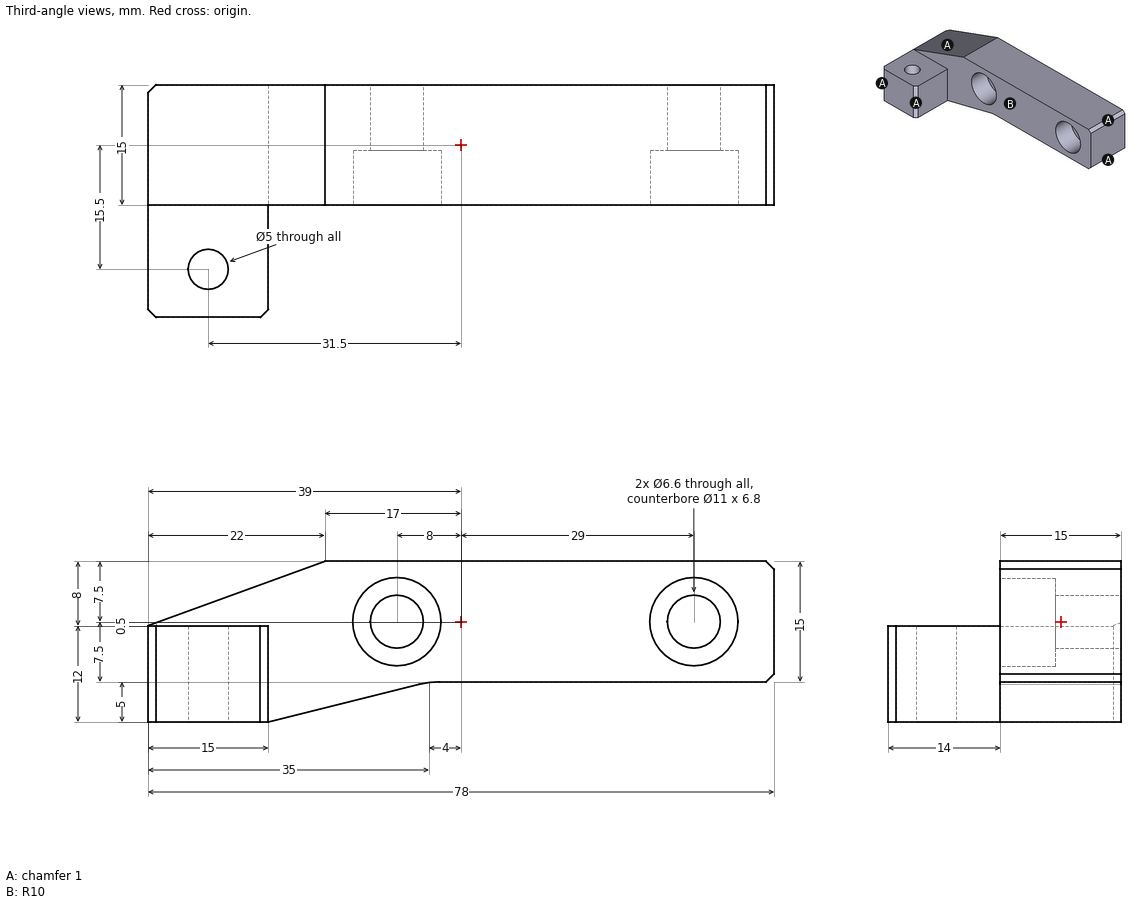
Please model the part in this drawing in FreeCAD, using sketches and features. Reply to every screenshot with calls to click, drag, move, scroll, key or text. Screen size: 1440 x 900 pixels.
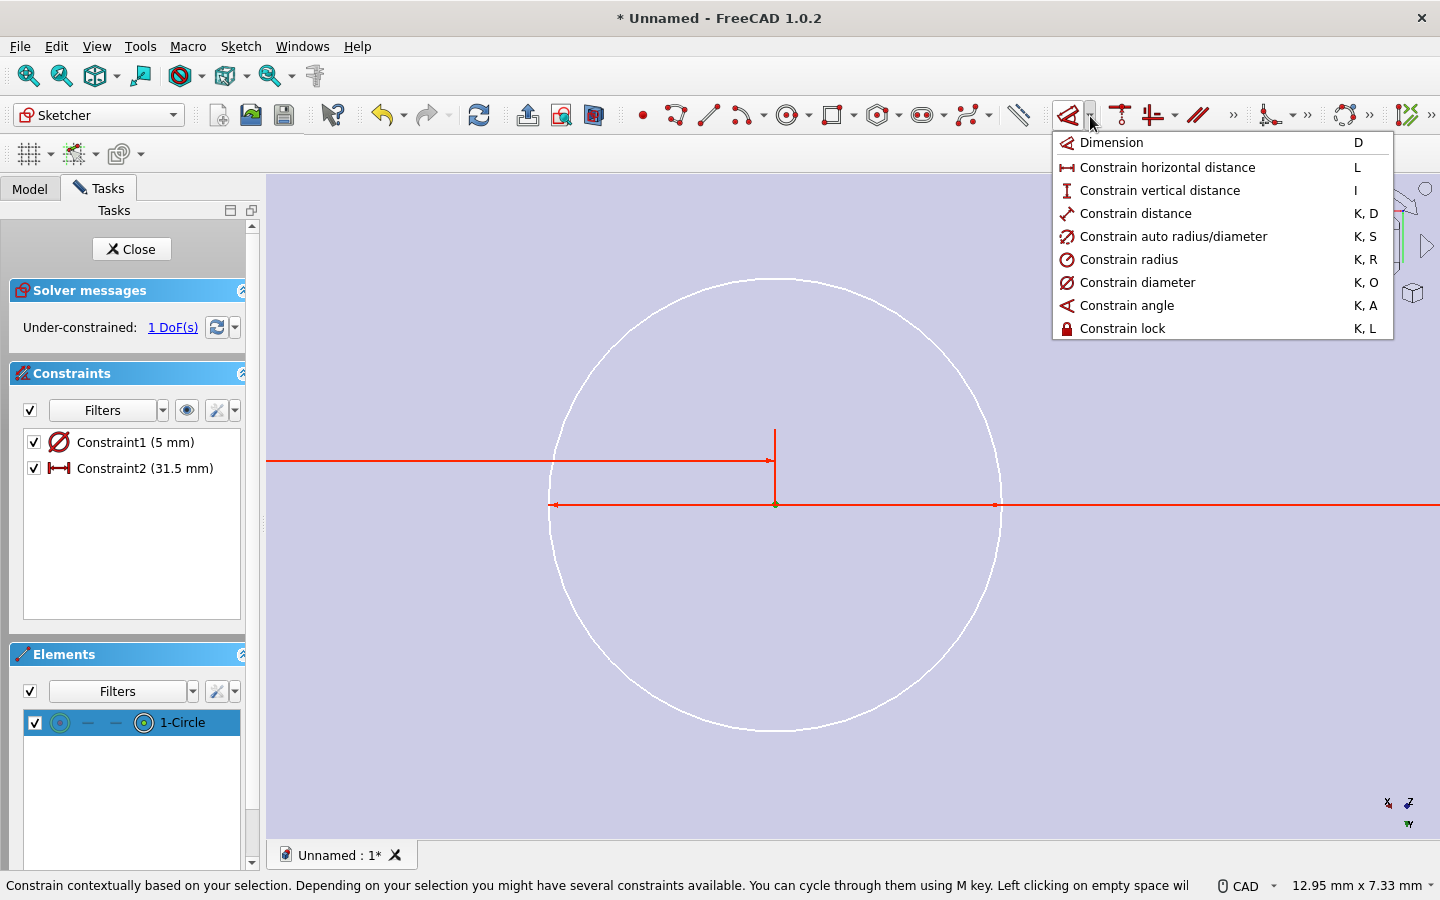
click(1223, 190)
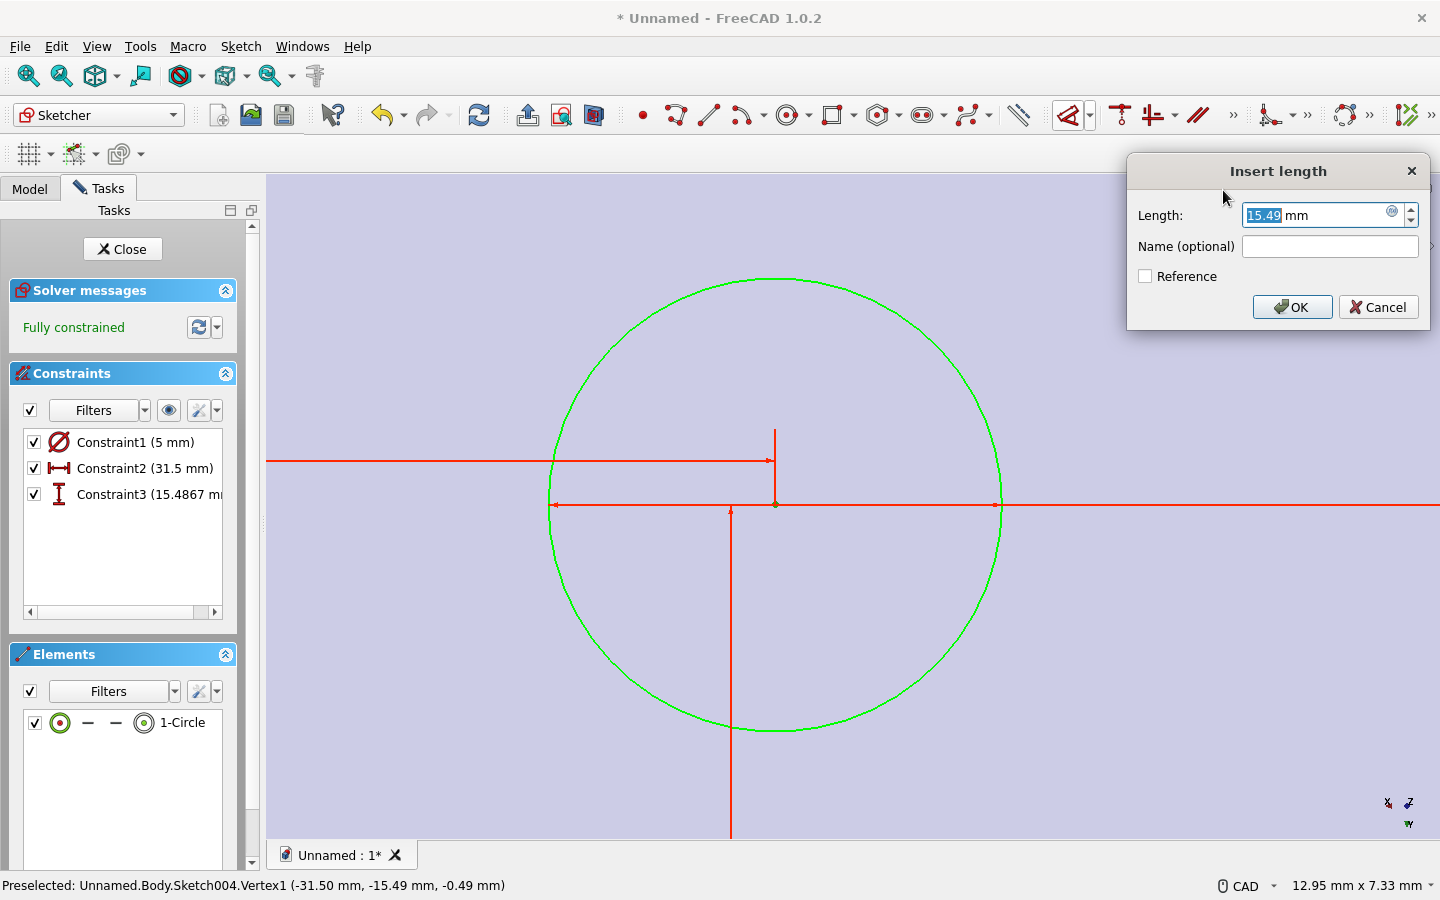
text(15.5)
key(Return)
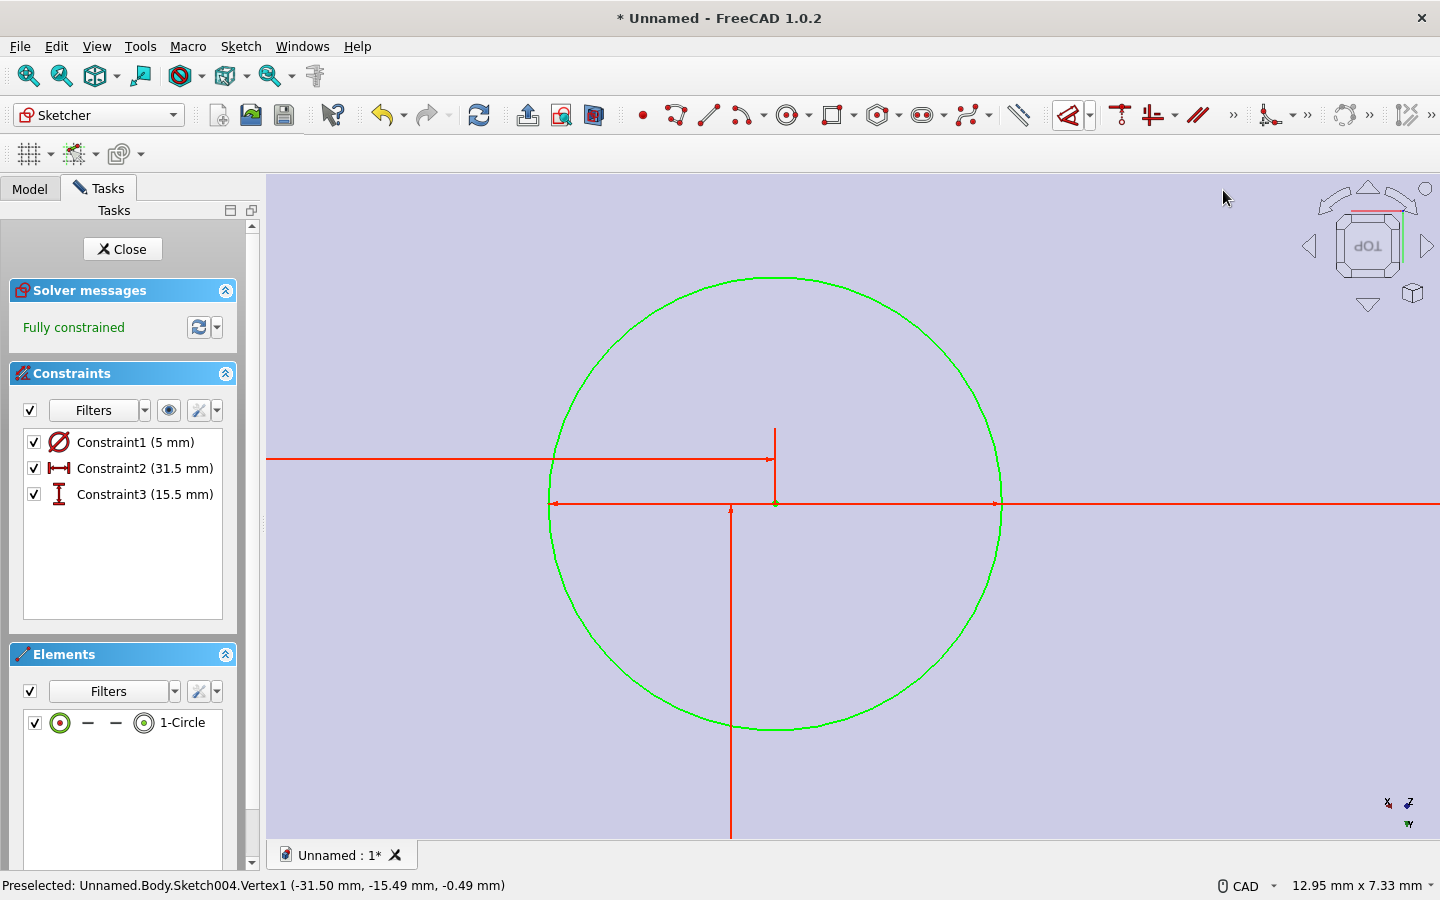
click(123, 249)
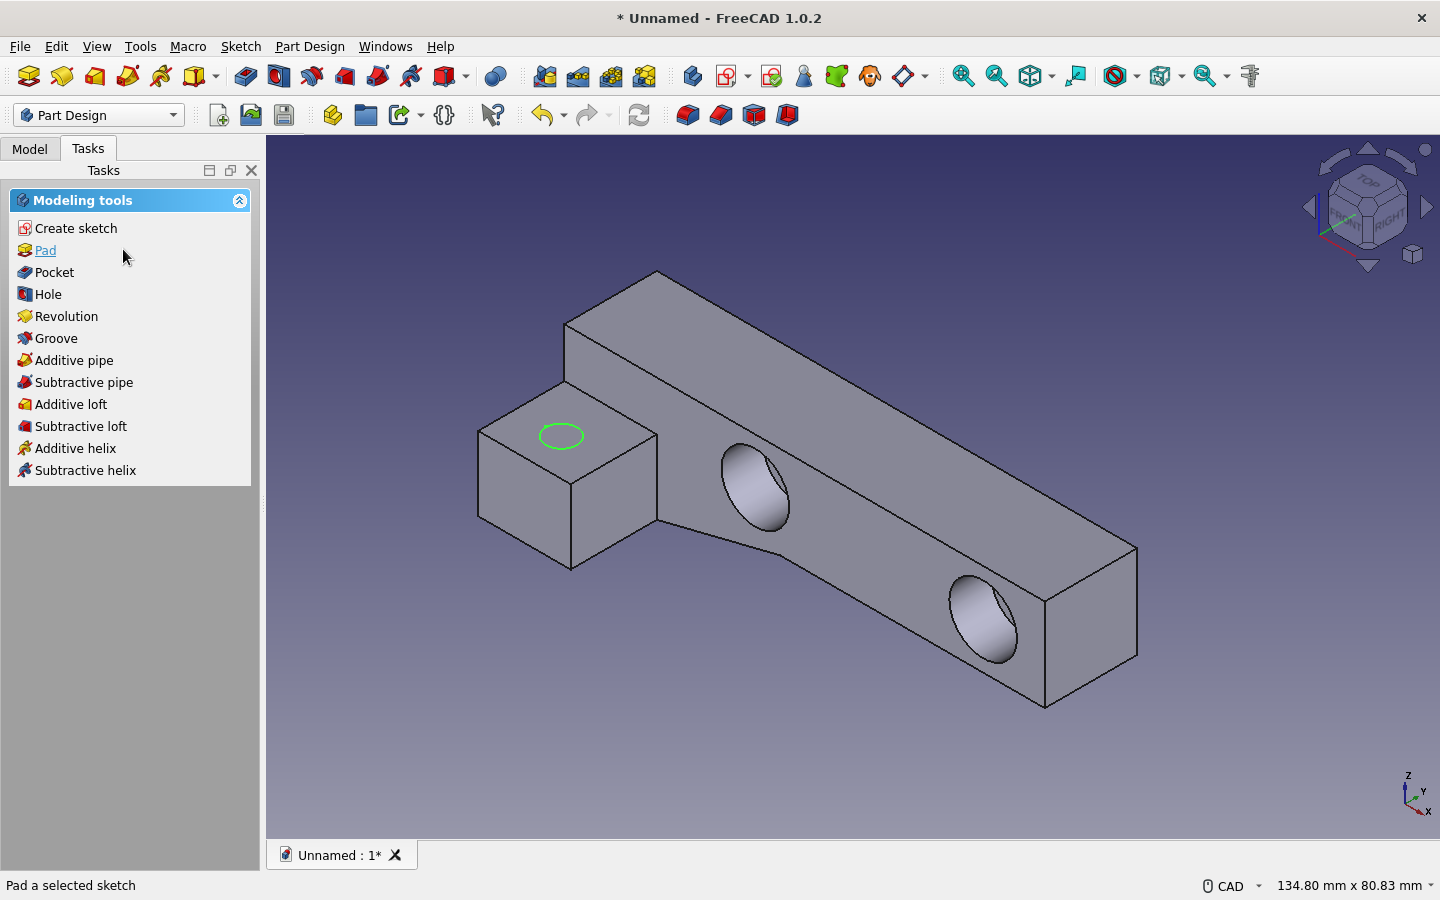
click(279, 76)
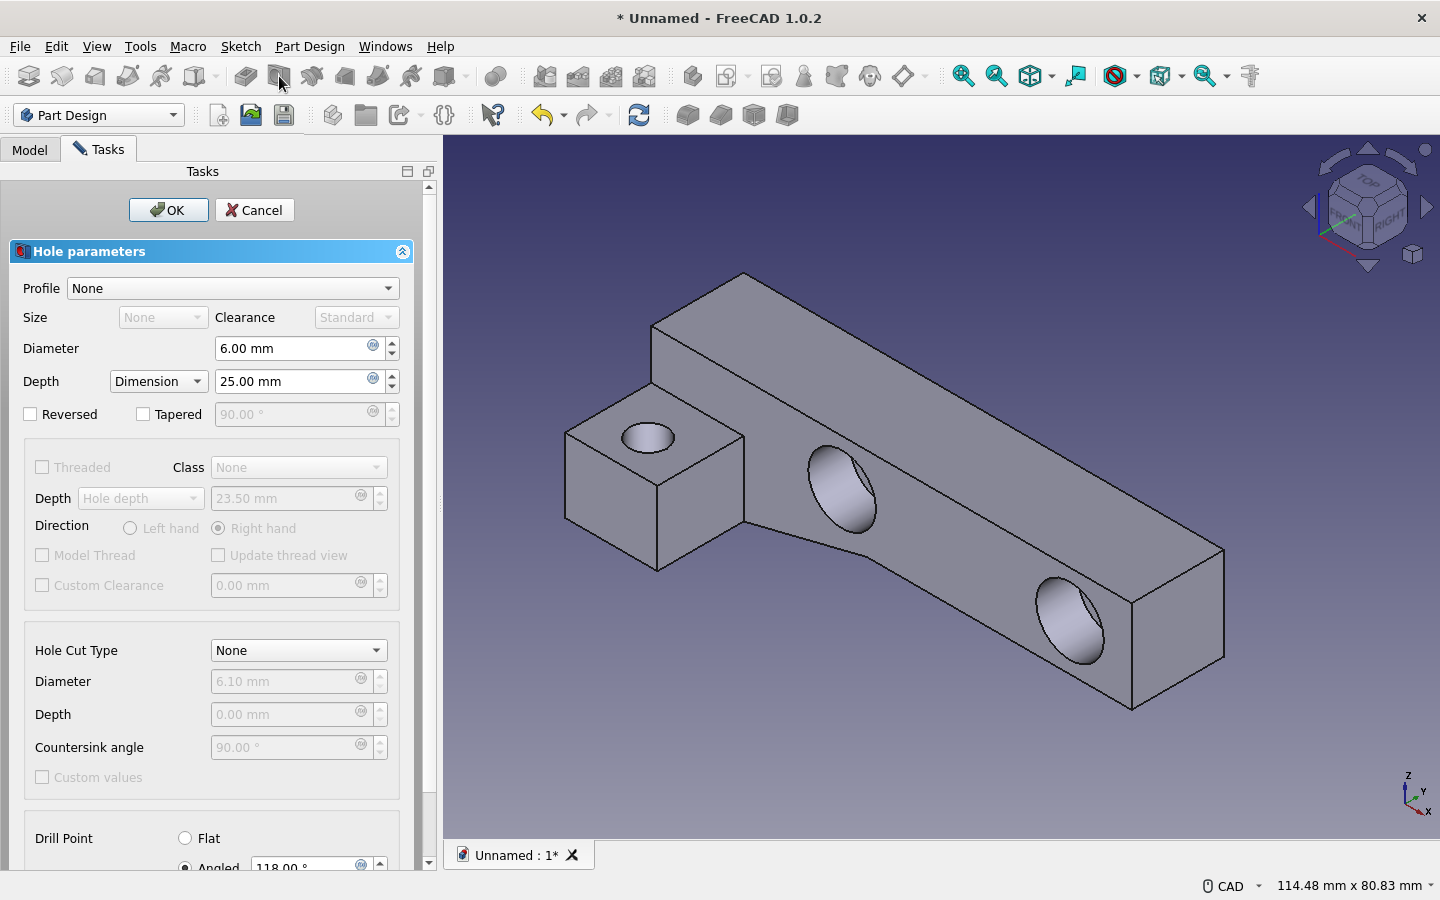
triple_click(300, 348)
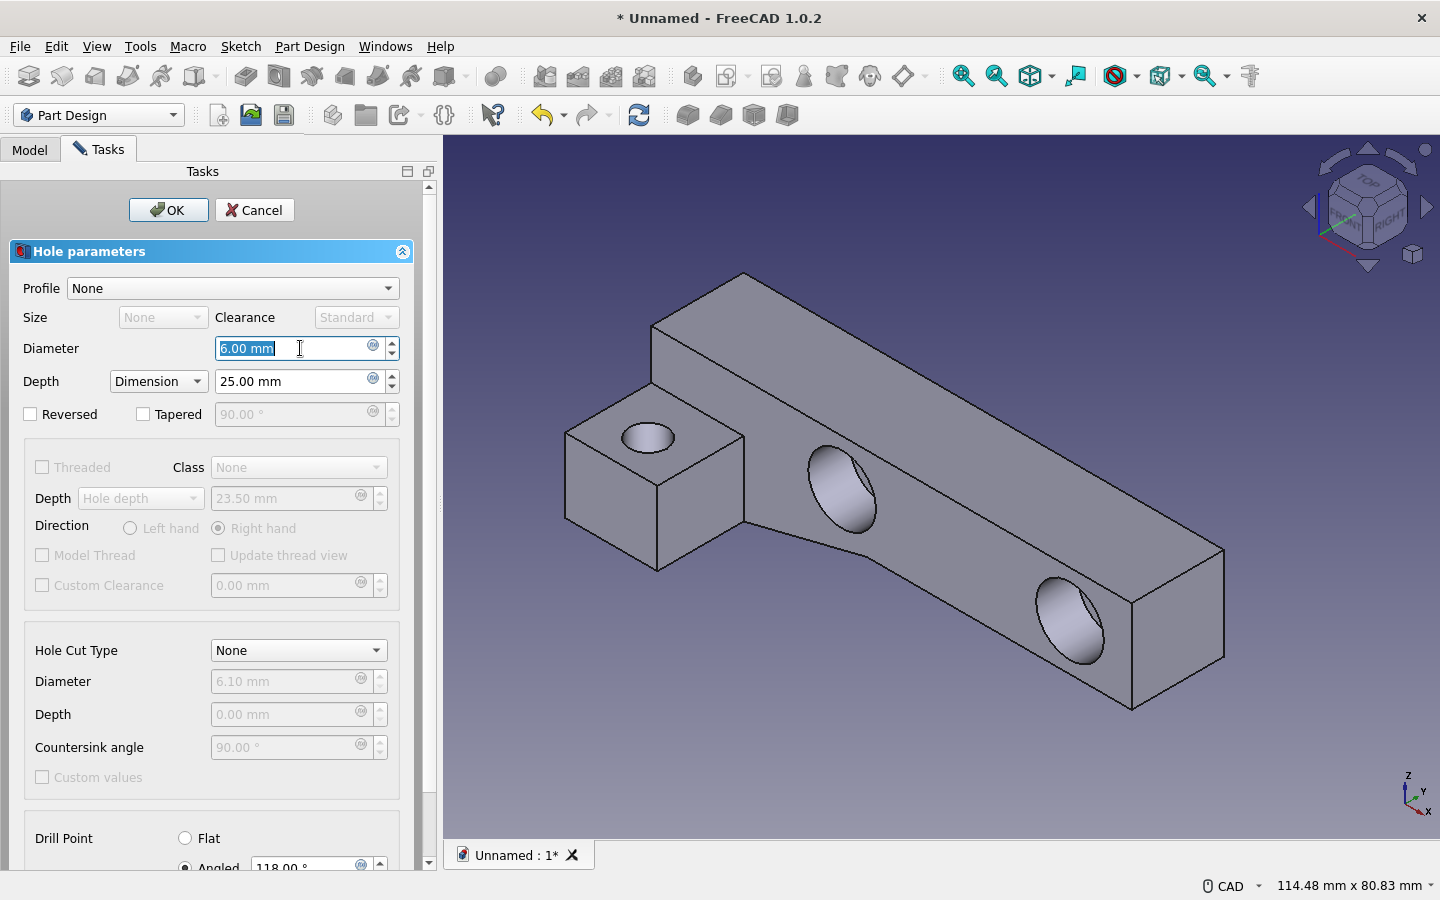
text(5)
key(Tab)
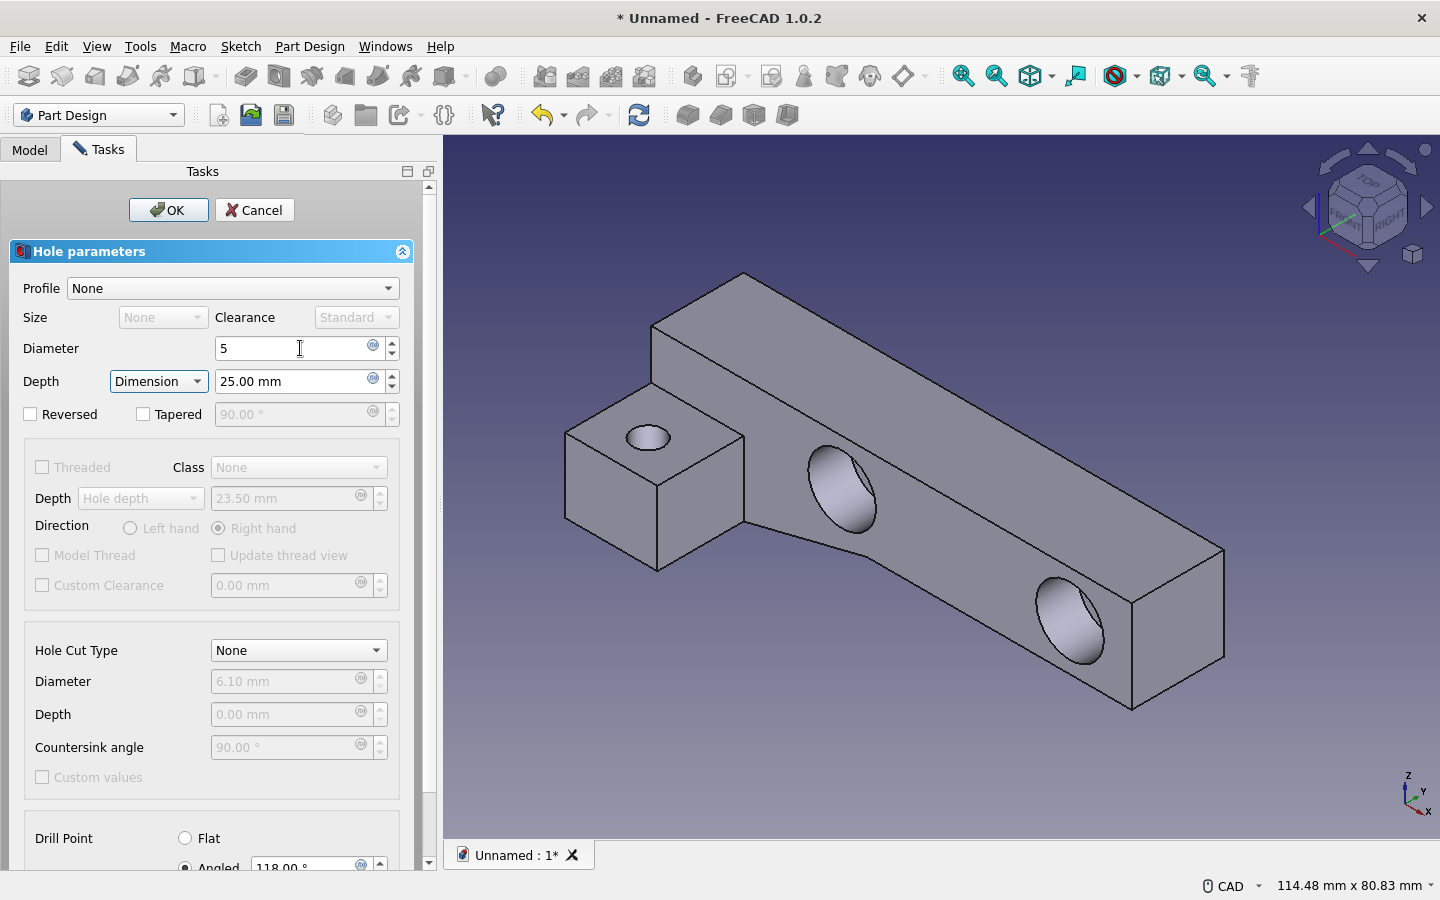
click(160, 382)